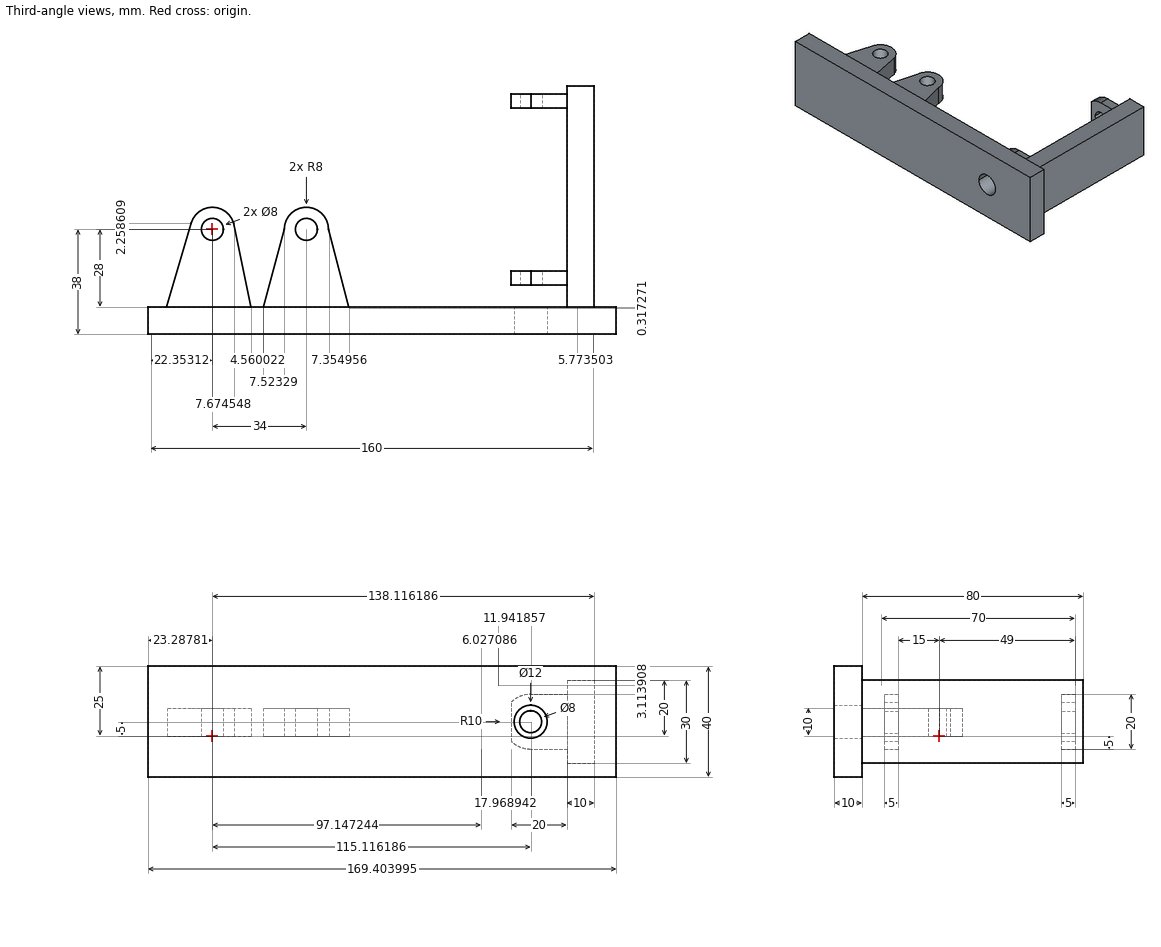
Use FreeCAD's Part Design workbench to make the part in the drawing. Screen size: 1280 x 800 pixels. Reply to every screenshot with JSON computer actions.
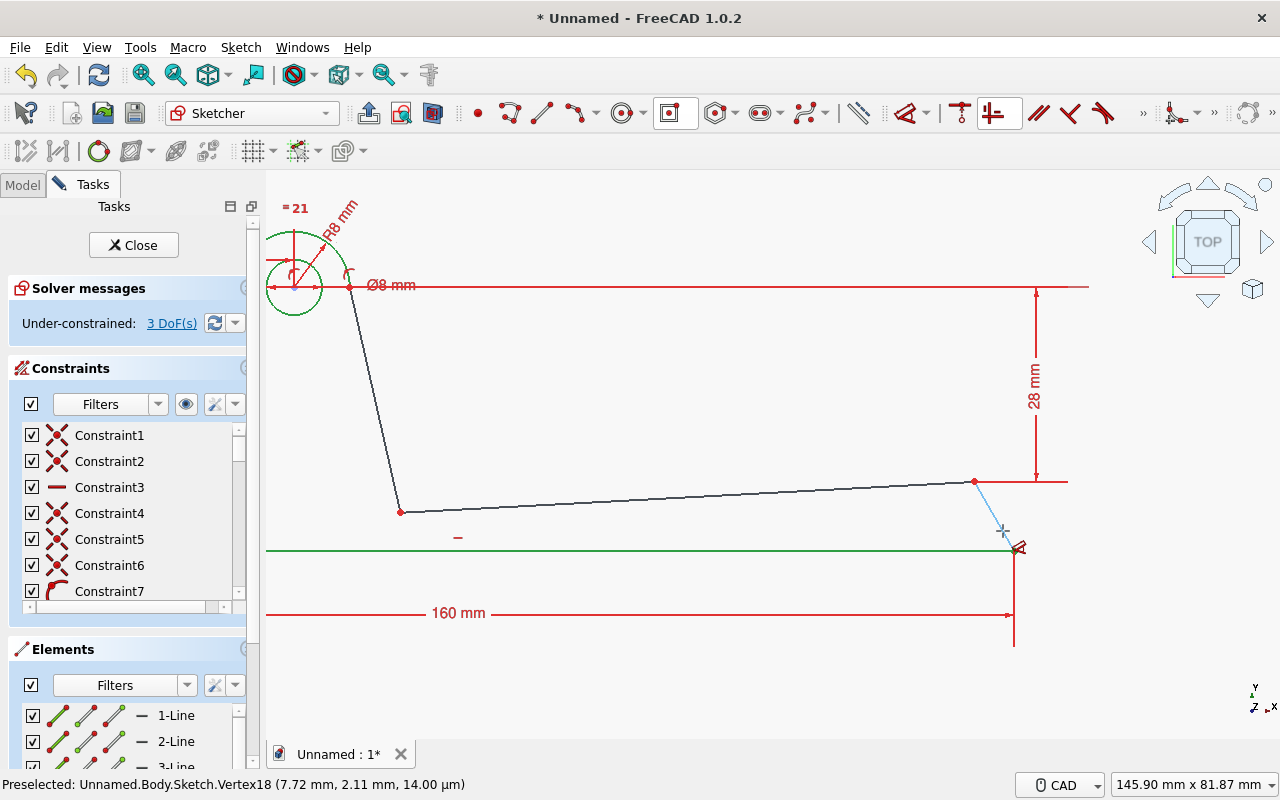
{"action": "left_click", "coordinate": [1002, 531]}
{"action": "left_click", "coordinate": [994, 585]}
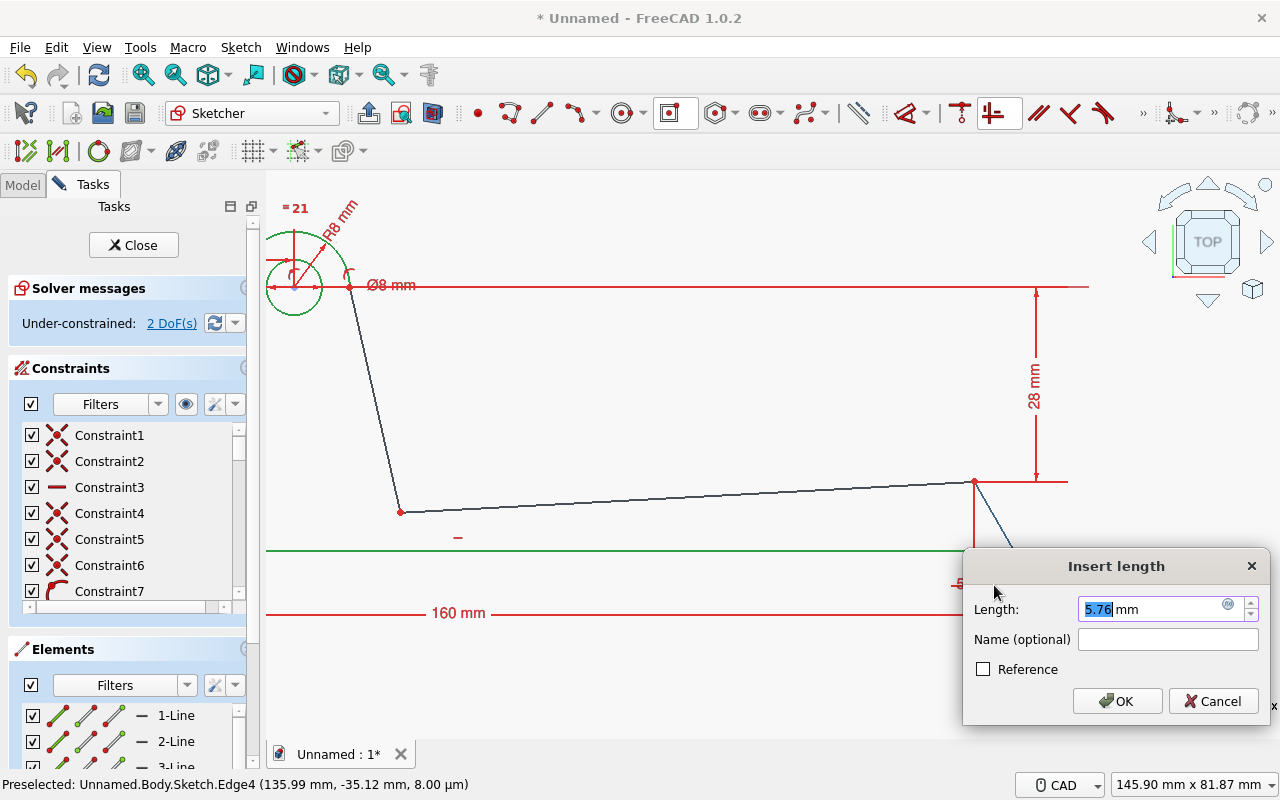
{"action": "type", "text": "5.773503"}
{"action": "key", "text": "Return"}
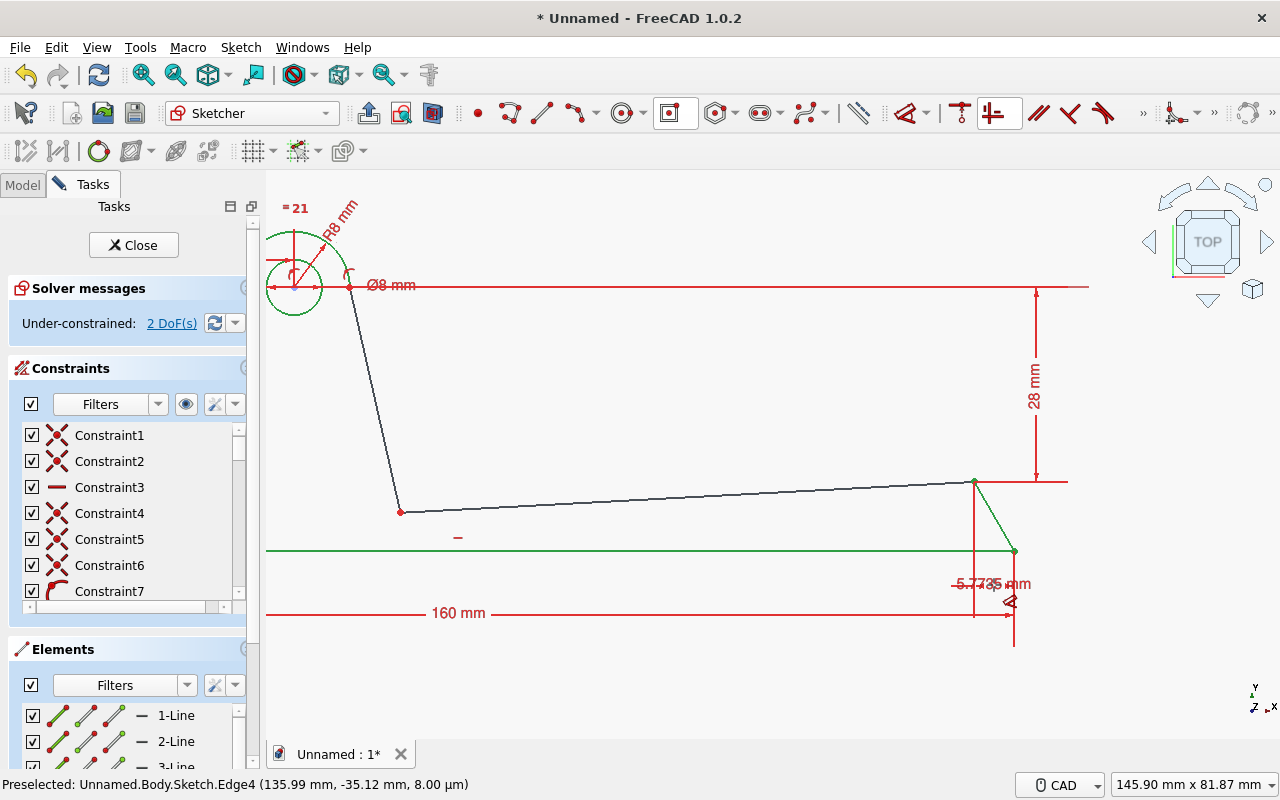
{"action": "scroll", "coordinate": [802, 491], "scroll_direction": "up", "scroll_amount": 15}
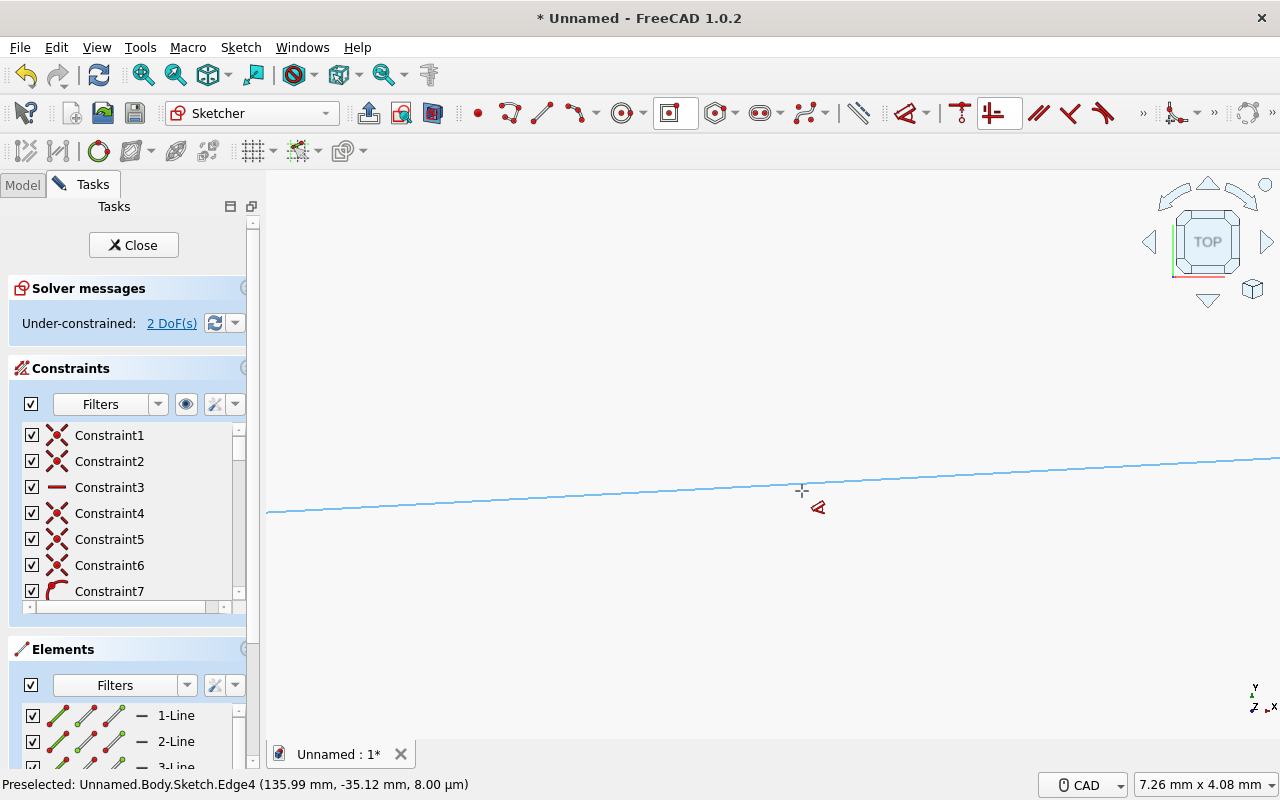
{"action": "left_click", "coordinate": [796, 484]}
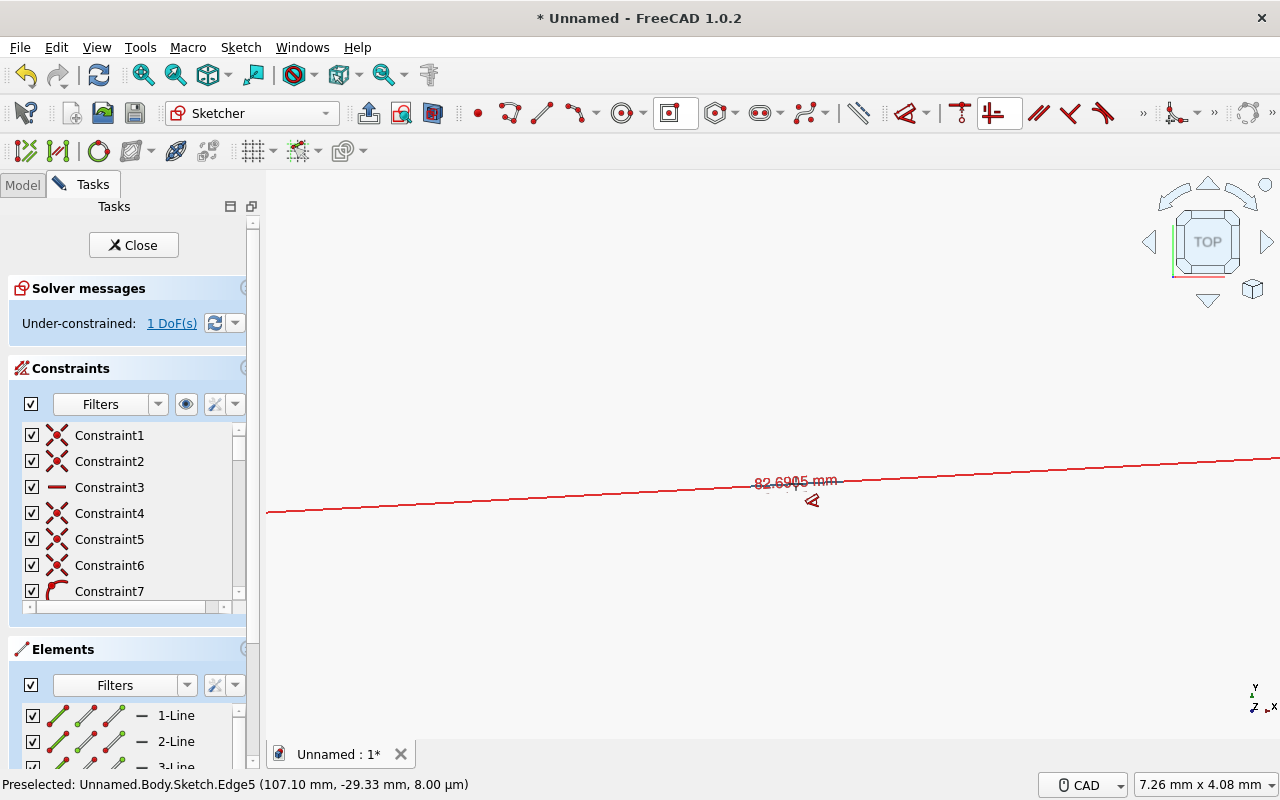
{"action": "key", "text": "Escape"}
{"action": "key", "text": "Escape"}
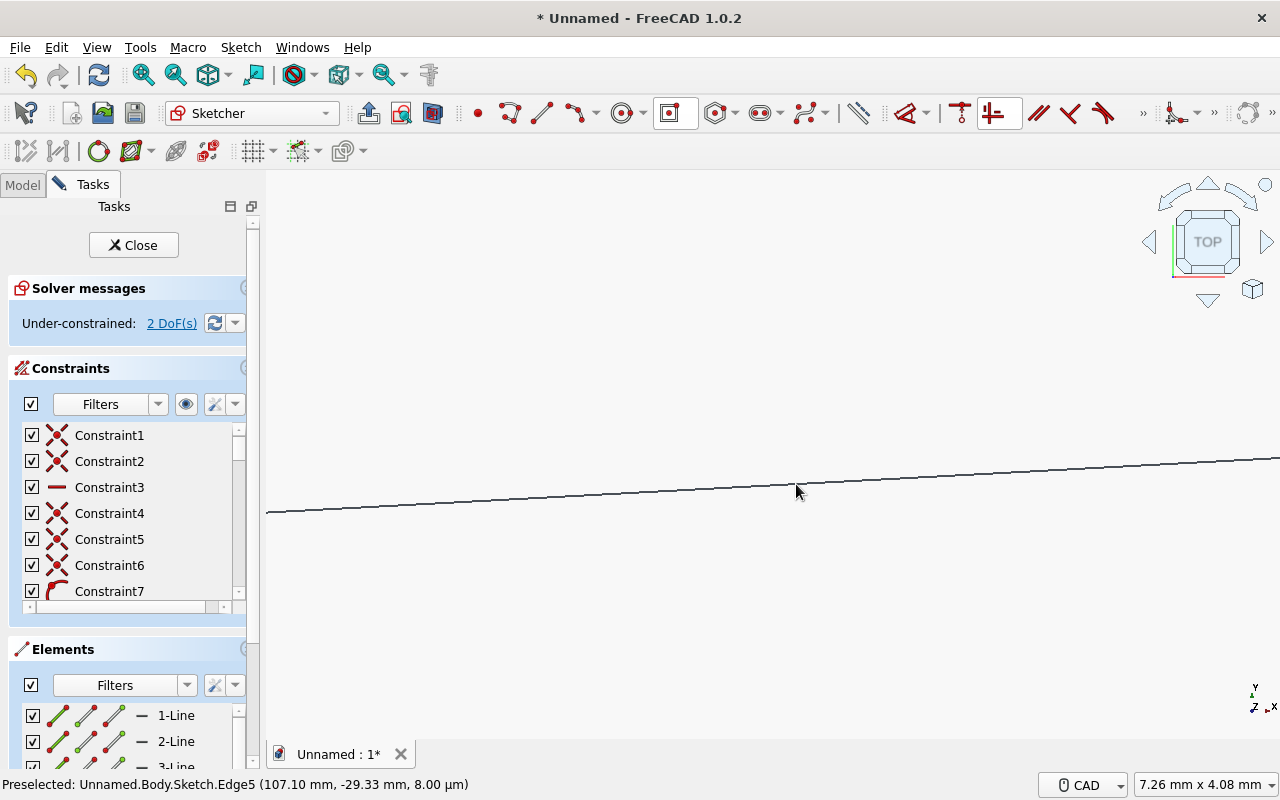
{"action": "left_click", "coordinate": [796, 484]}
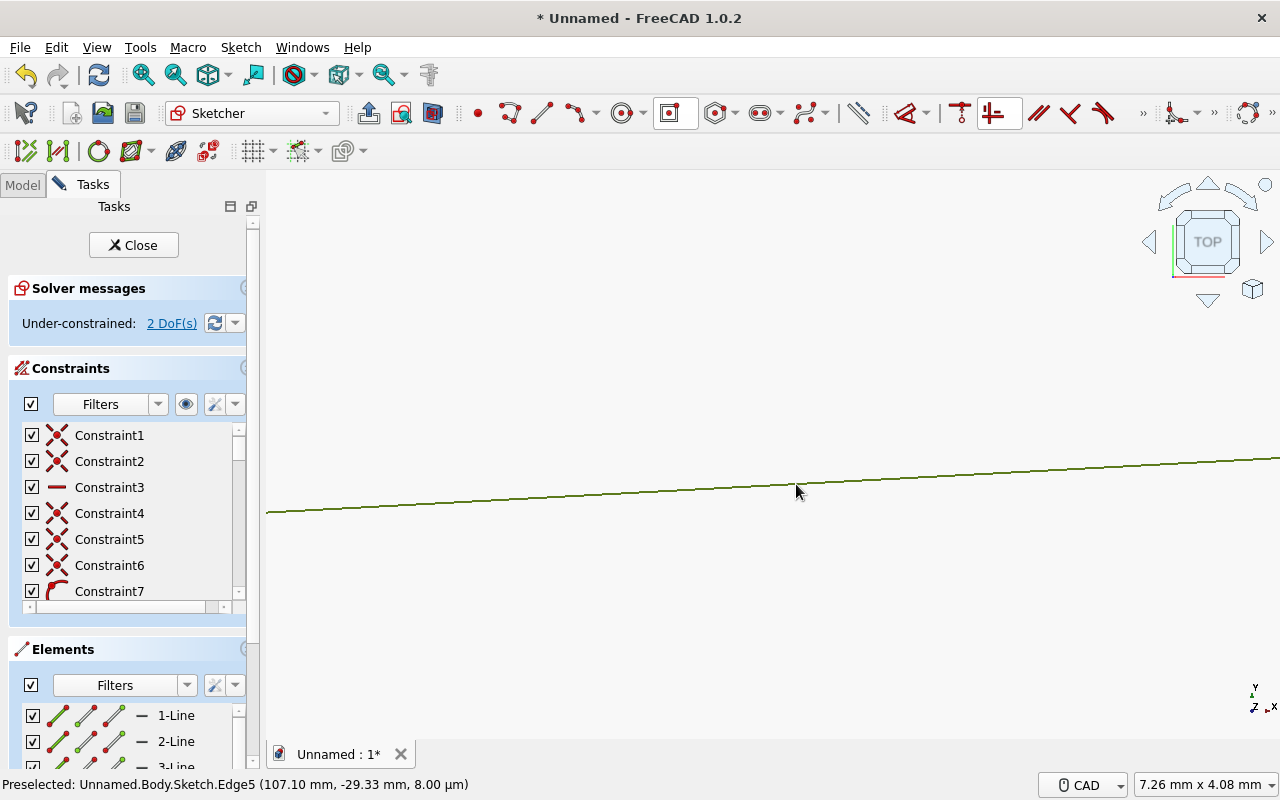
{"action": "left_click", "coordinate": [928, 114]}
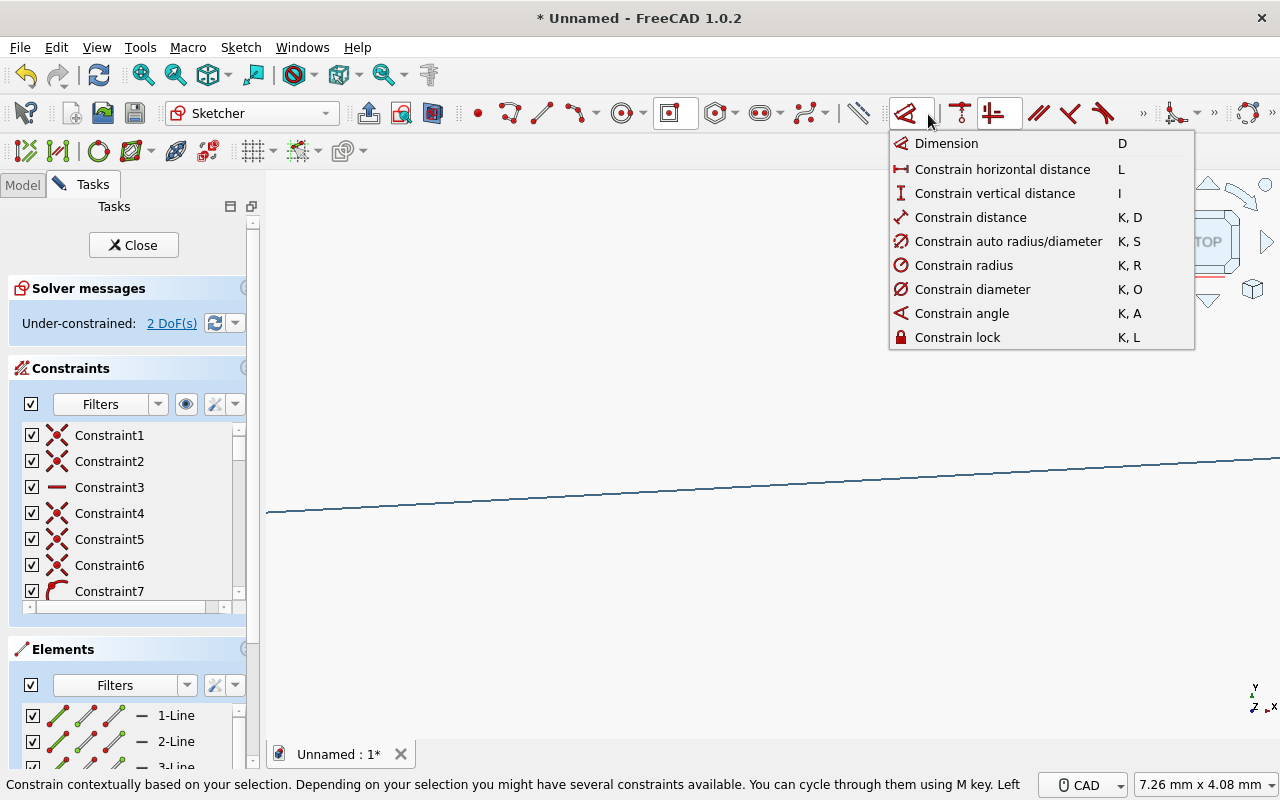
{"action": "left_click", "coordinate": [1042, 193]}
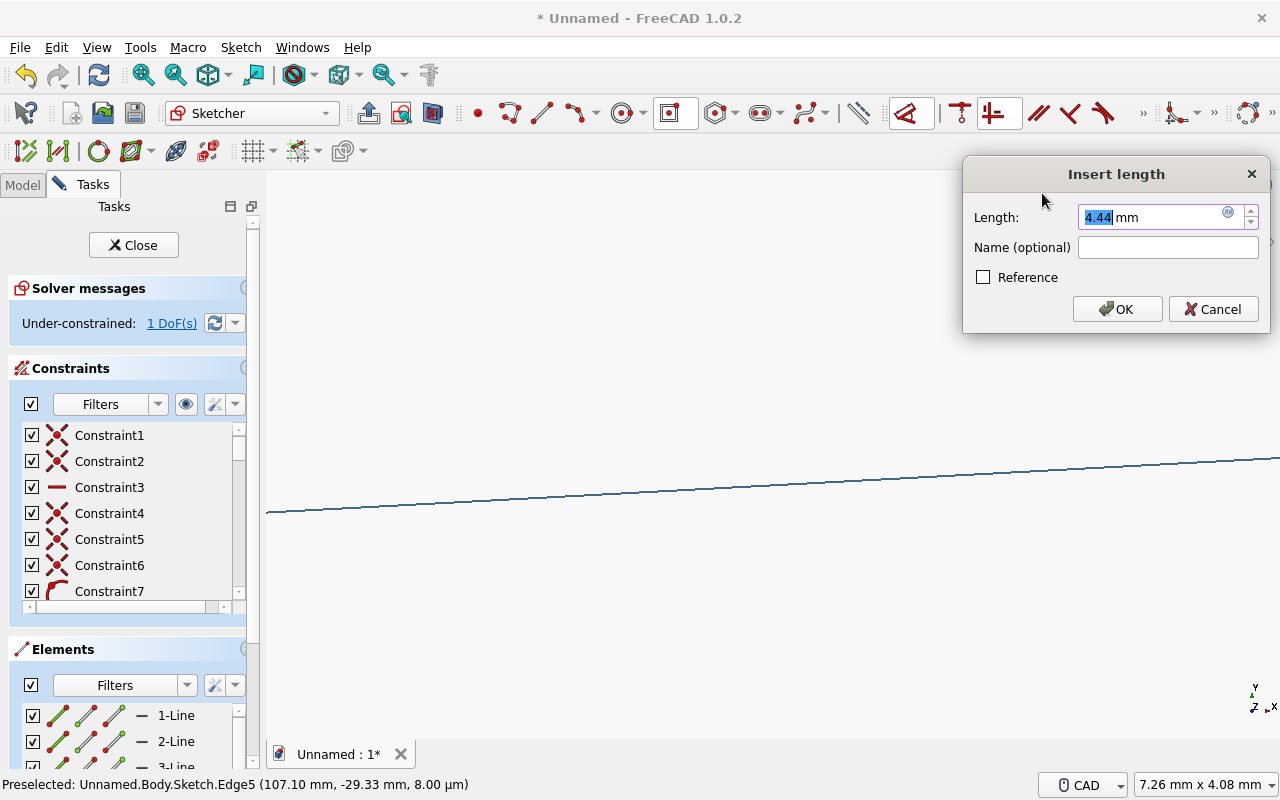
{"action": "type", "text": "0.317271"}
{"action": "key", "text": "Return"}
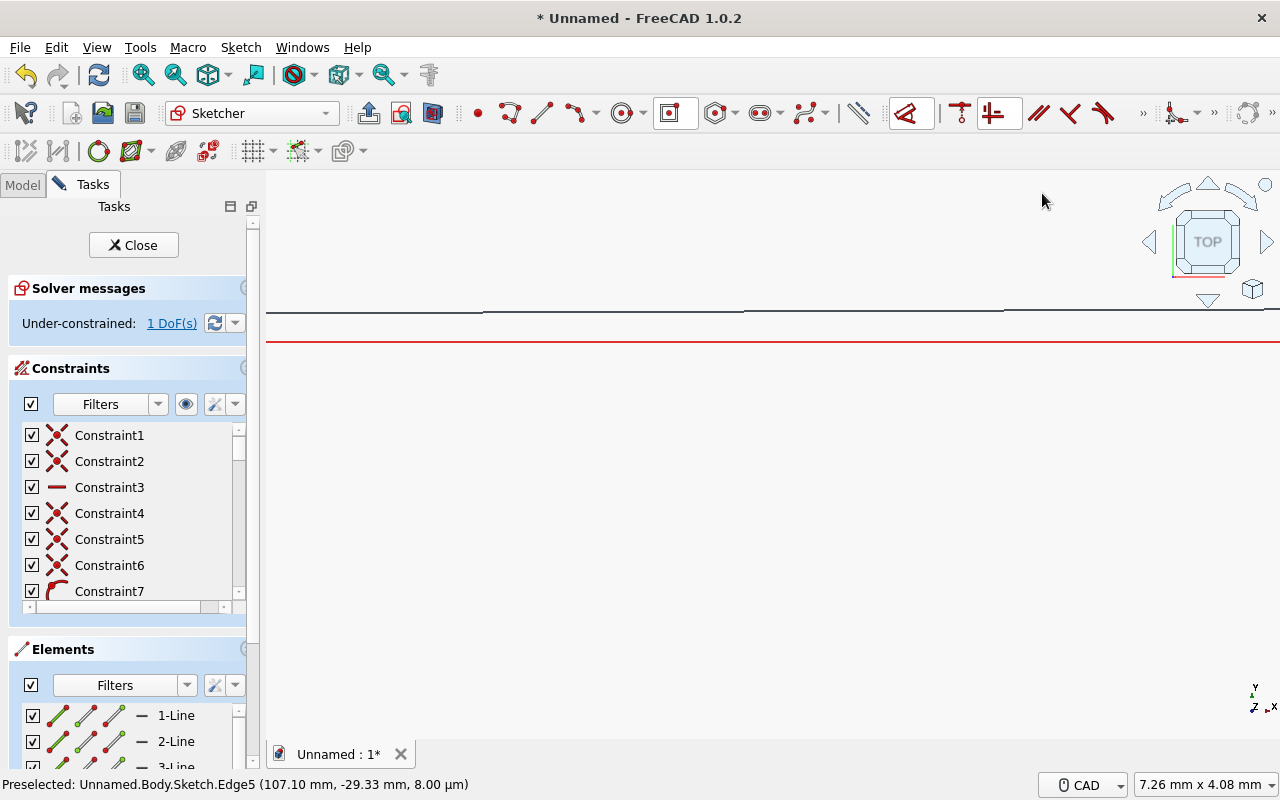
{"action": "scroll", "coordinate": [940, 523], "scroll_direction": "down", "scroll_amount": 17}